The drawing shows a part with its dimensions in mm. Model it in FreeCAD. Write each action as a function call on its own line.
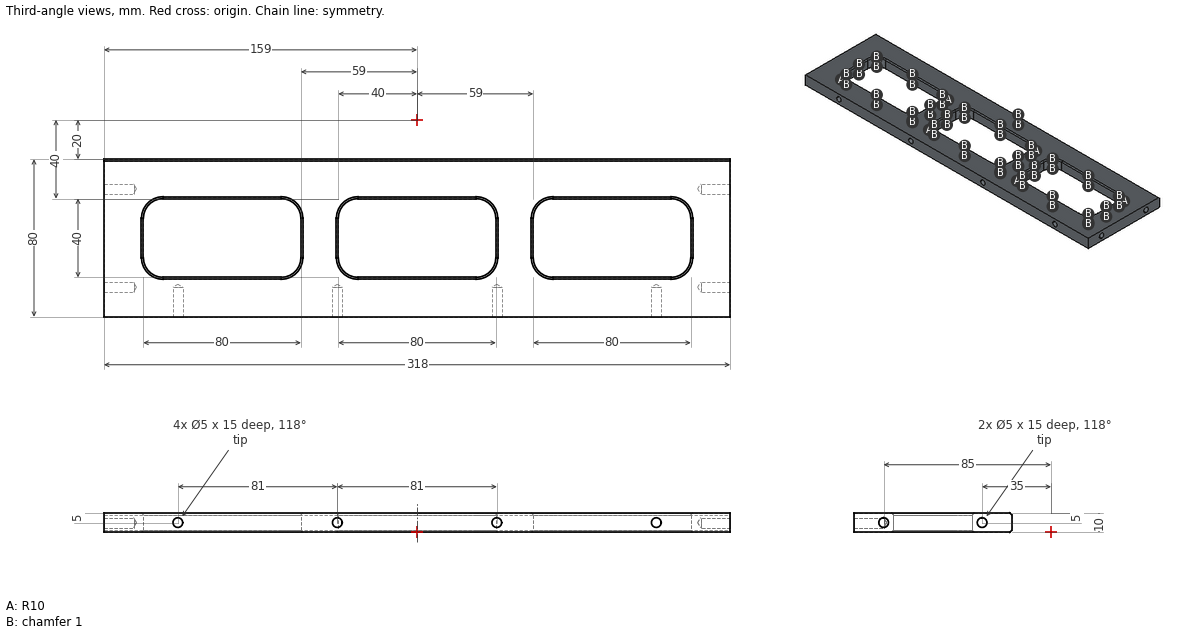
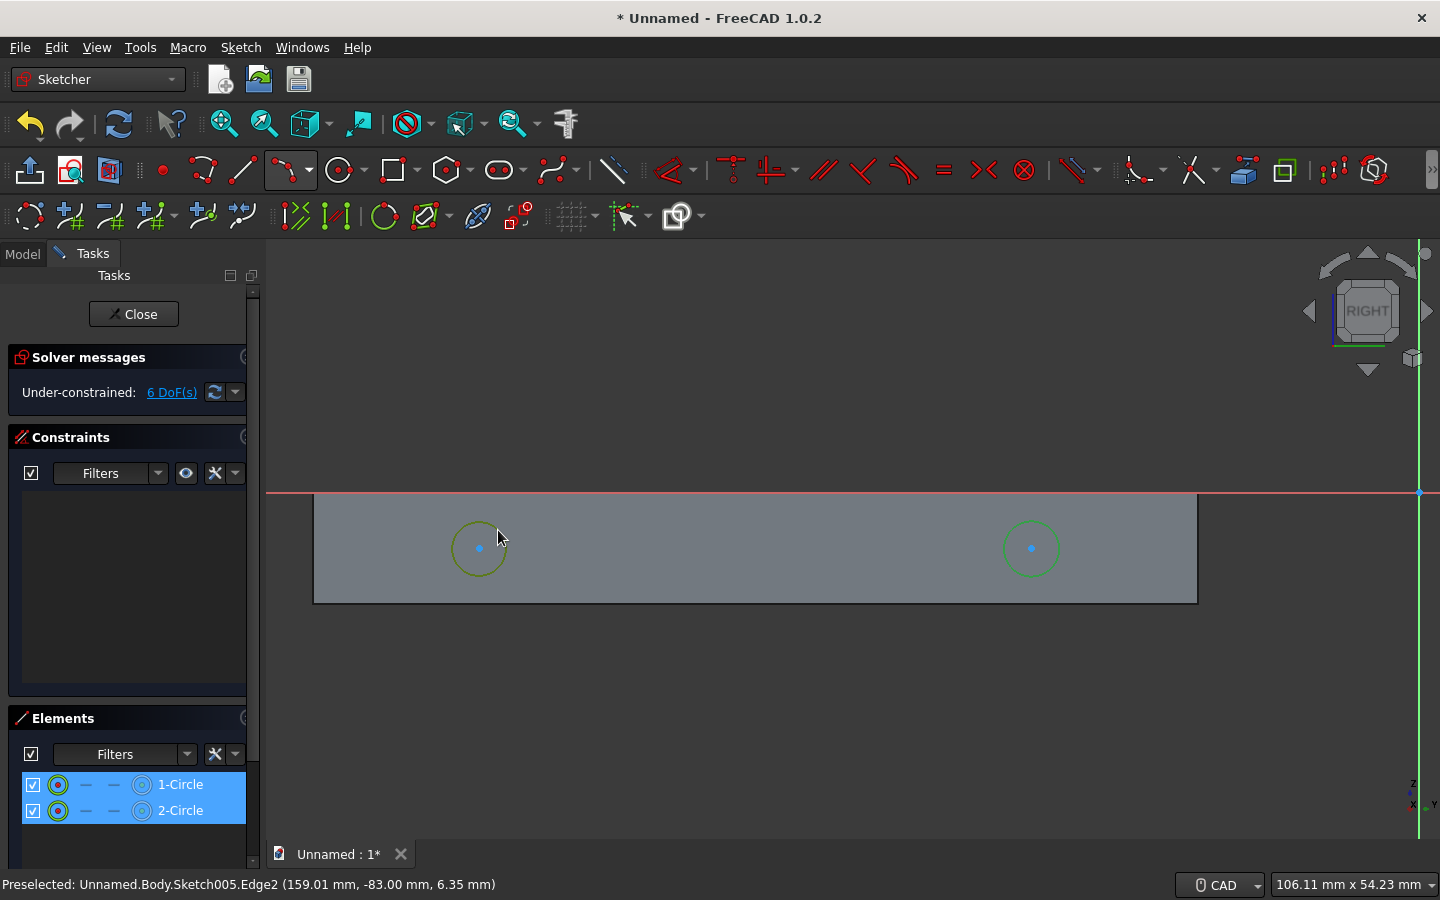
key(e)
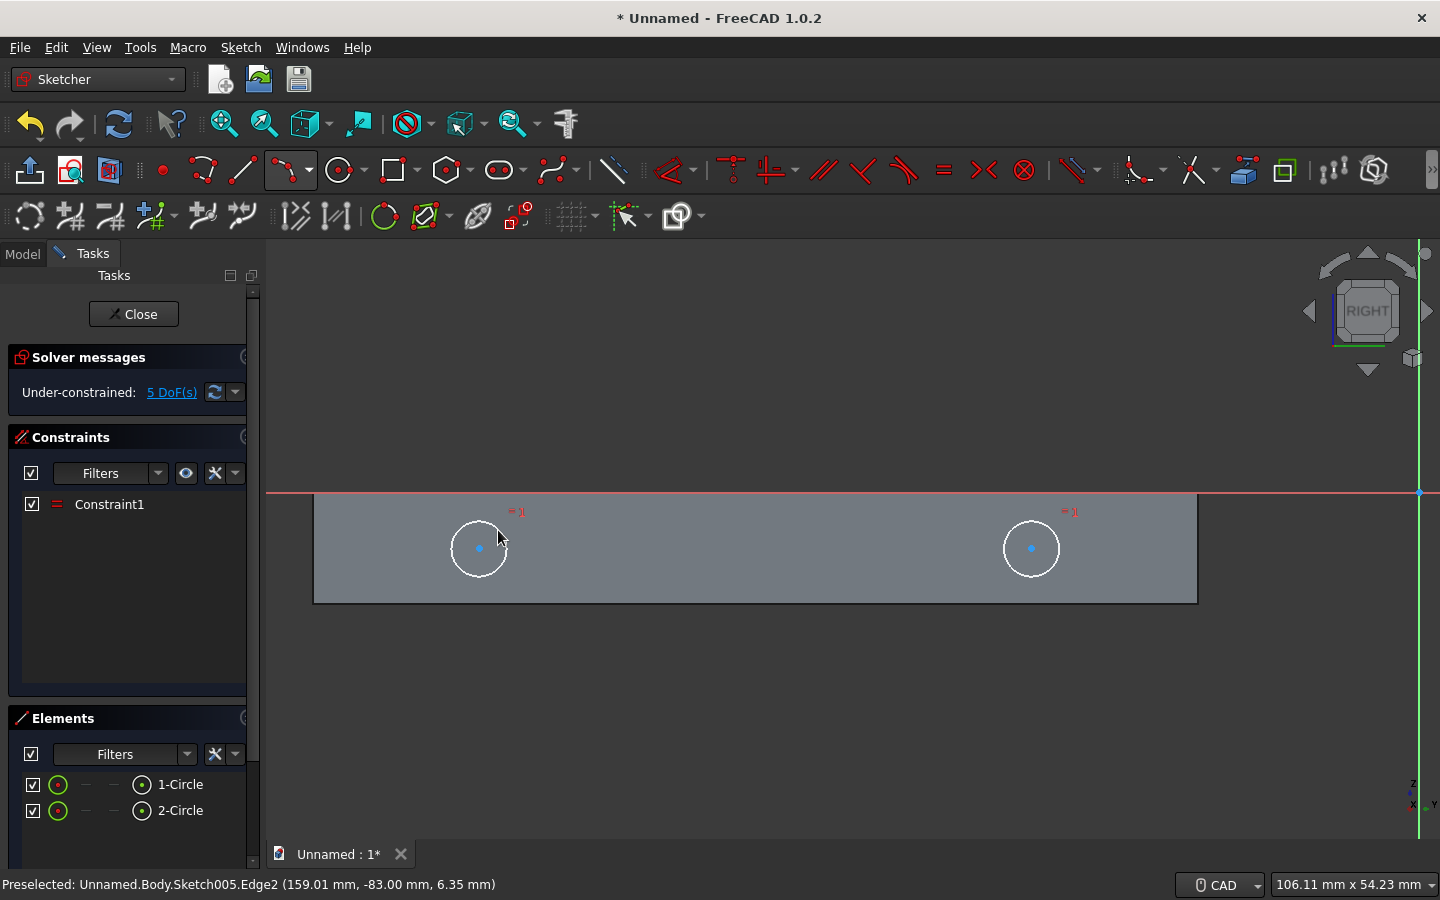
click(668, 170)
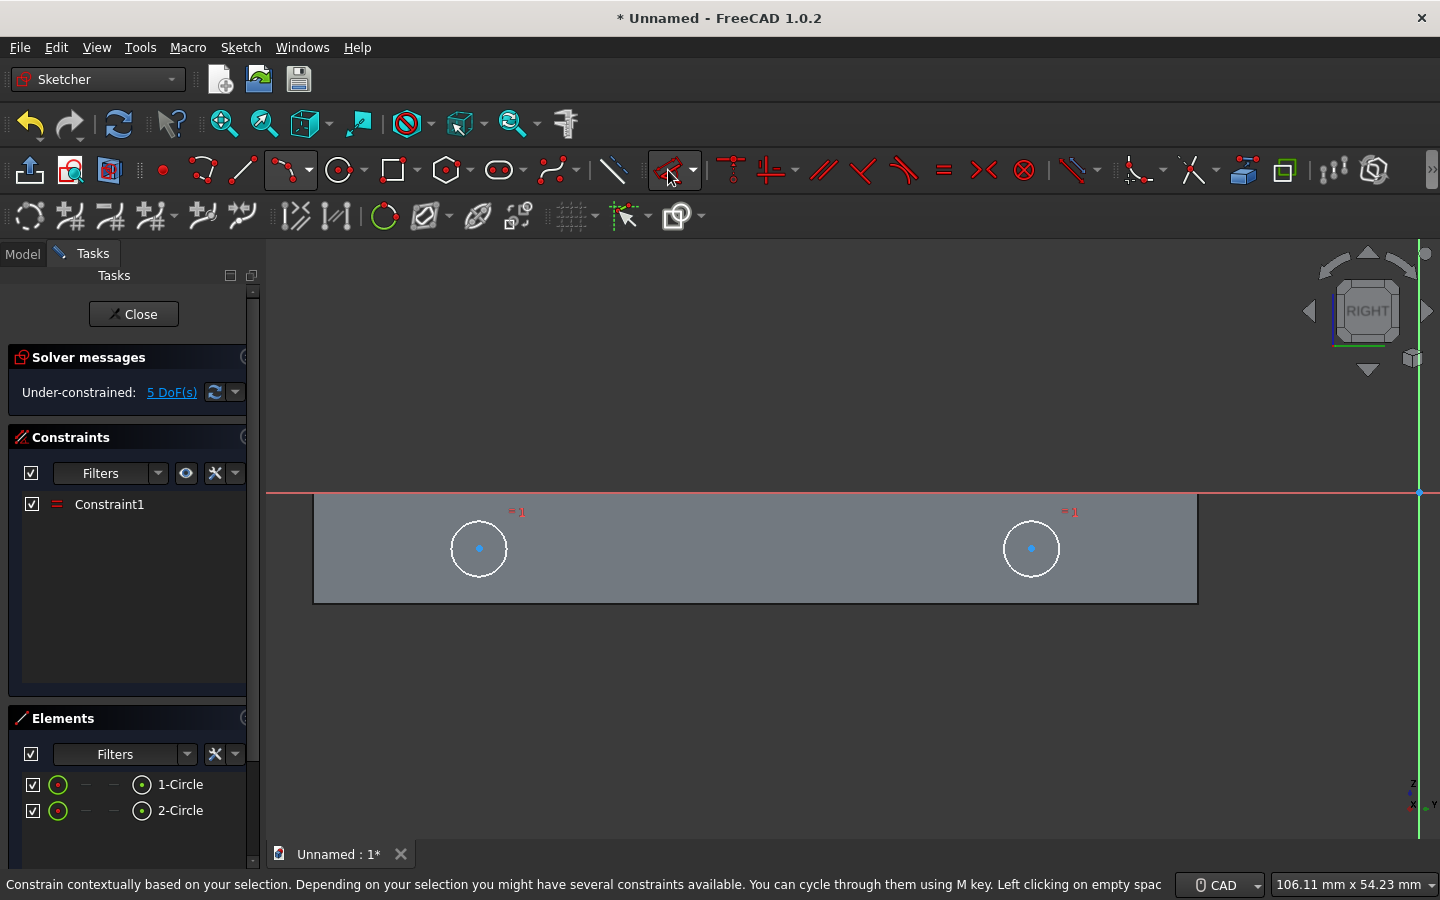
click(1051, 529)
click(1073, 506)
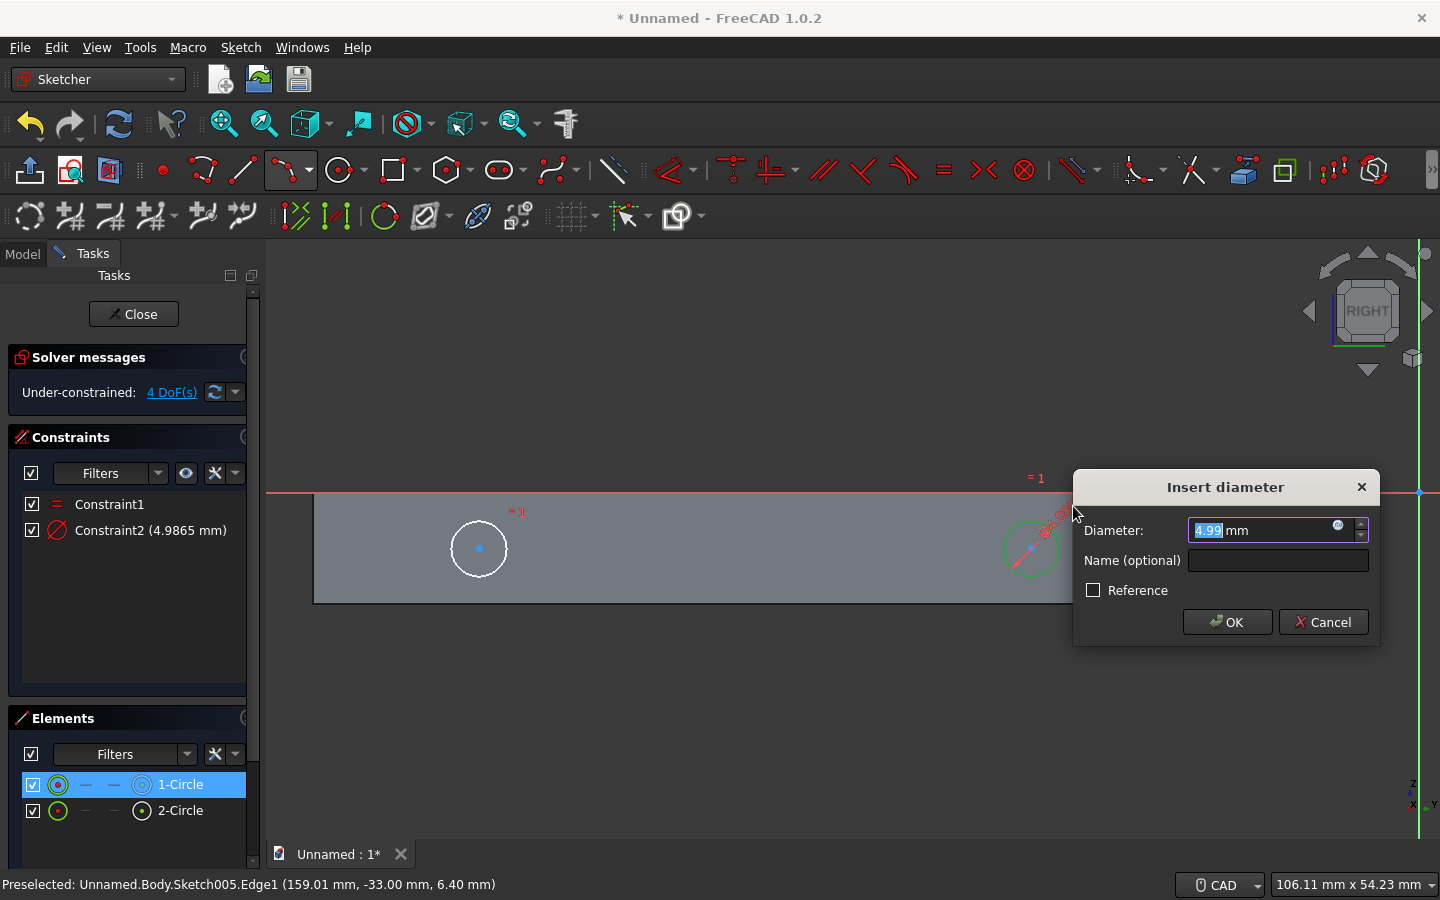
text(5)
key(Return)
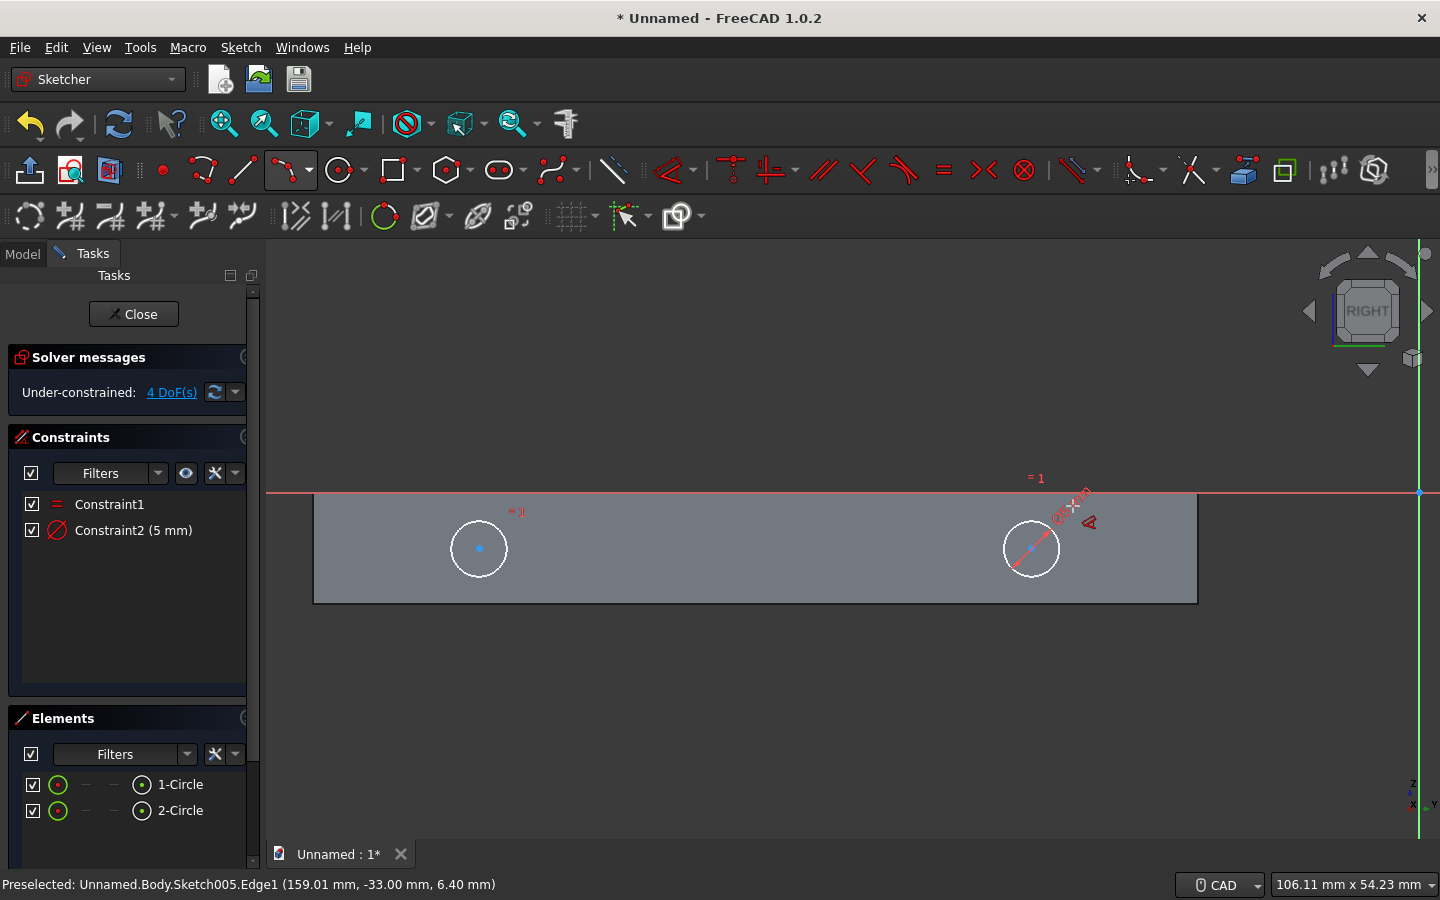
click(1032, 549)
click(998, 521)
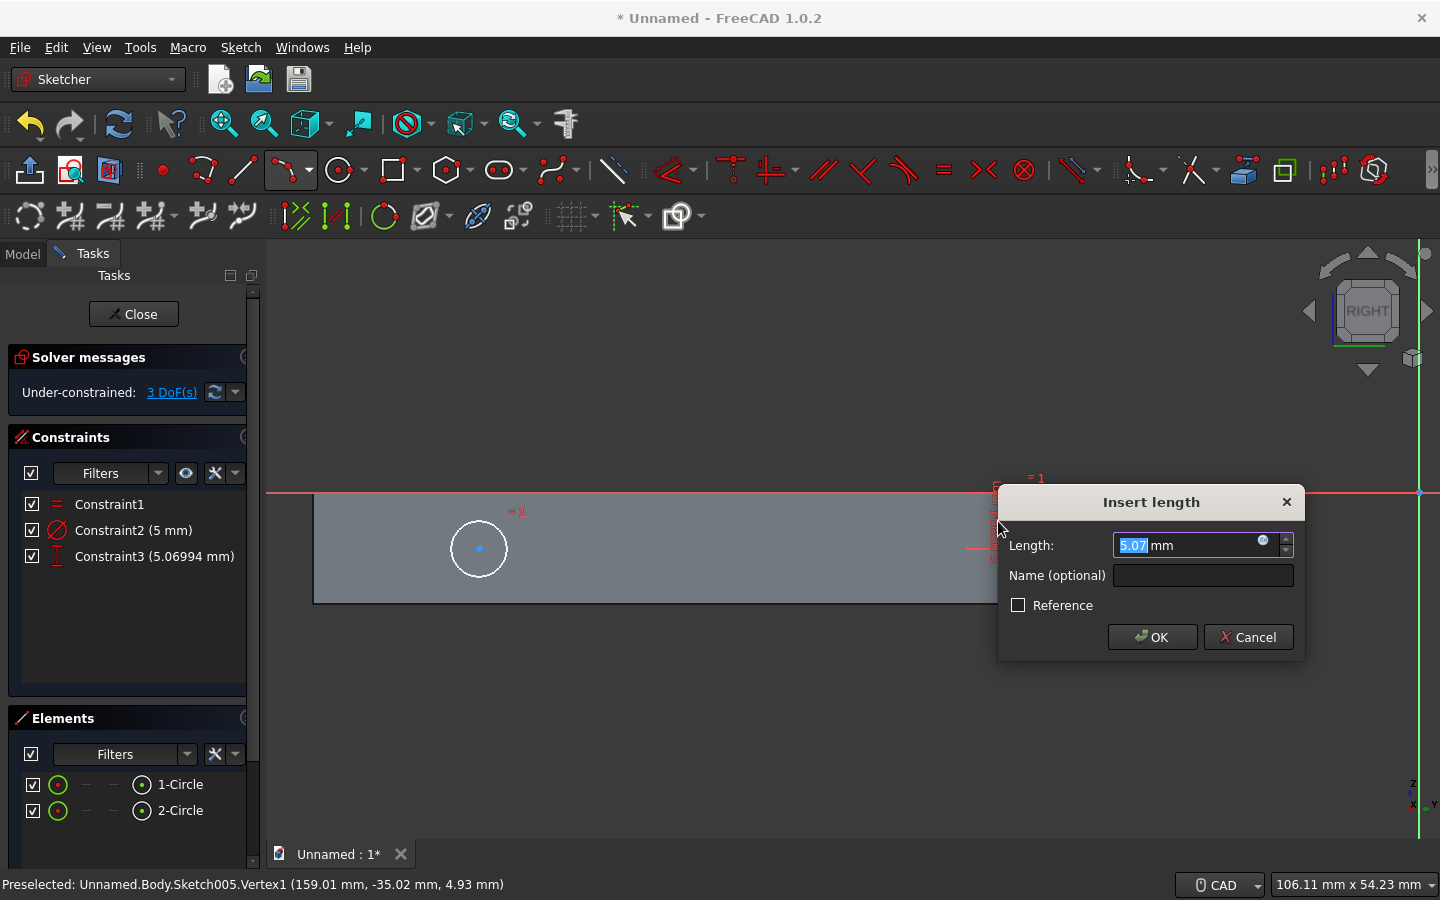
text(5)
key(Return)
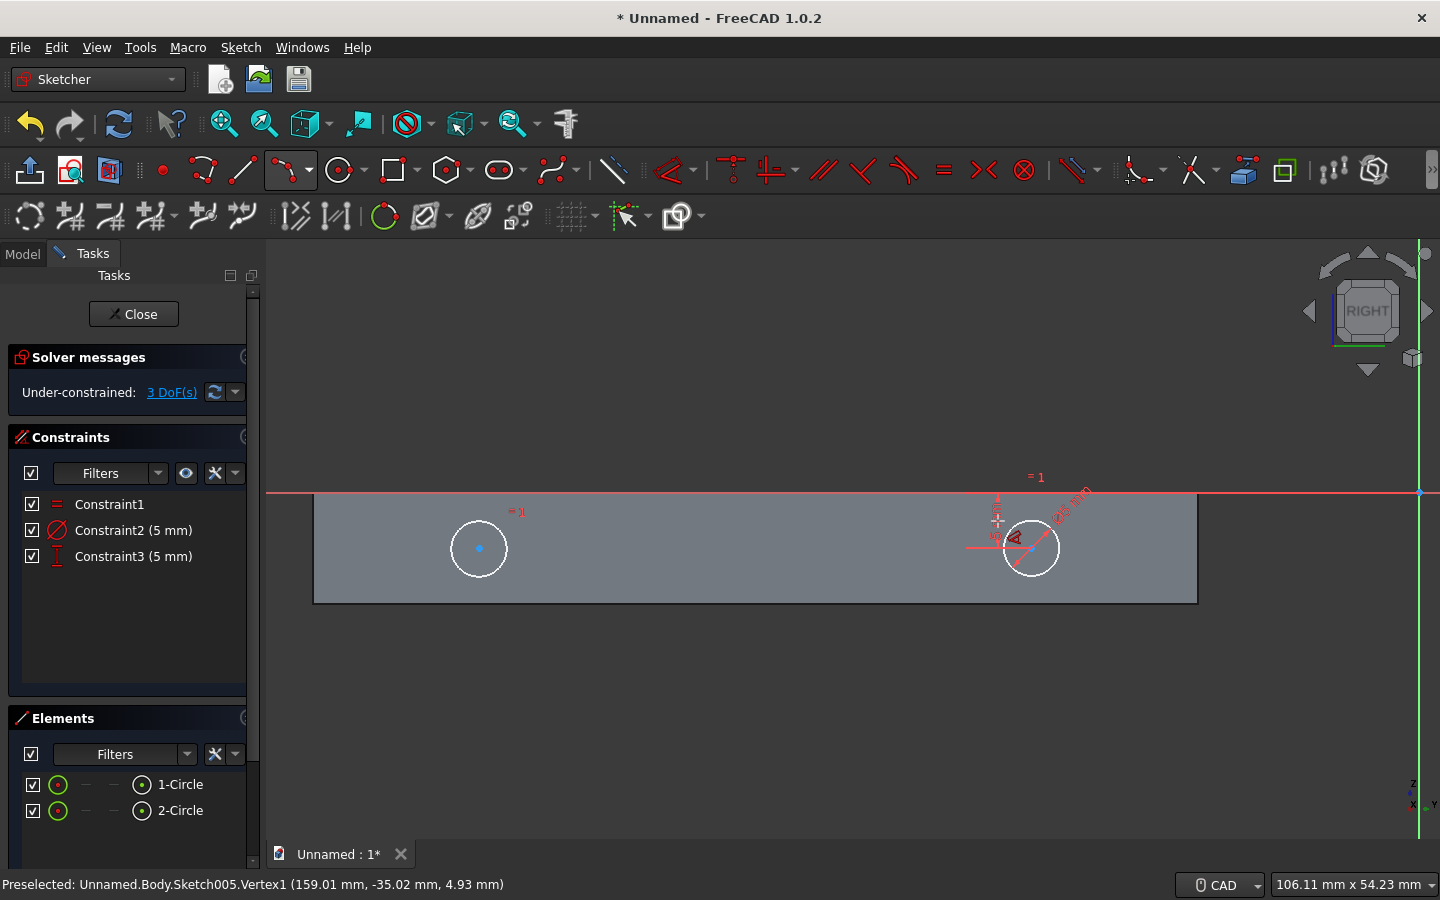
click(479, 549)
click(445, 521)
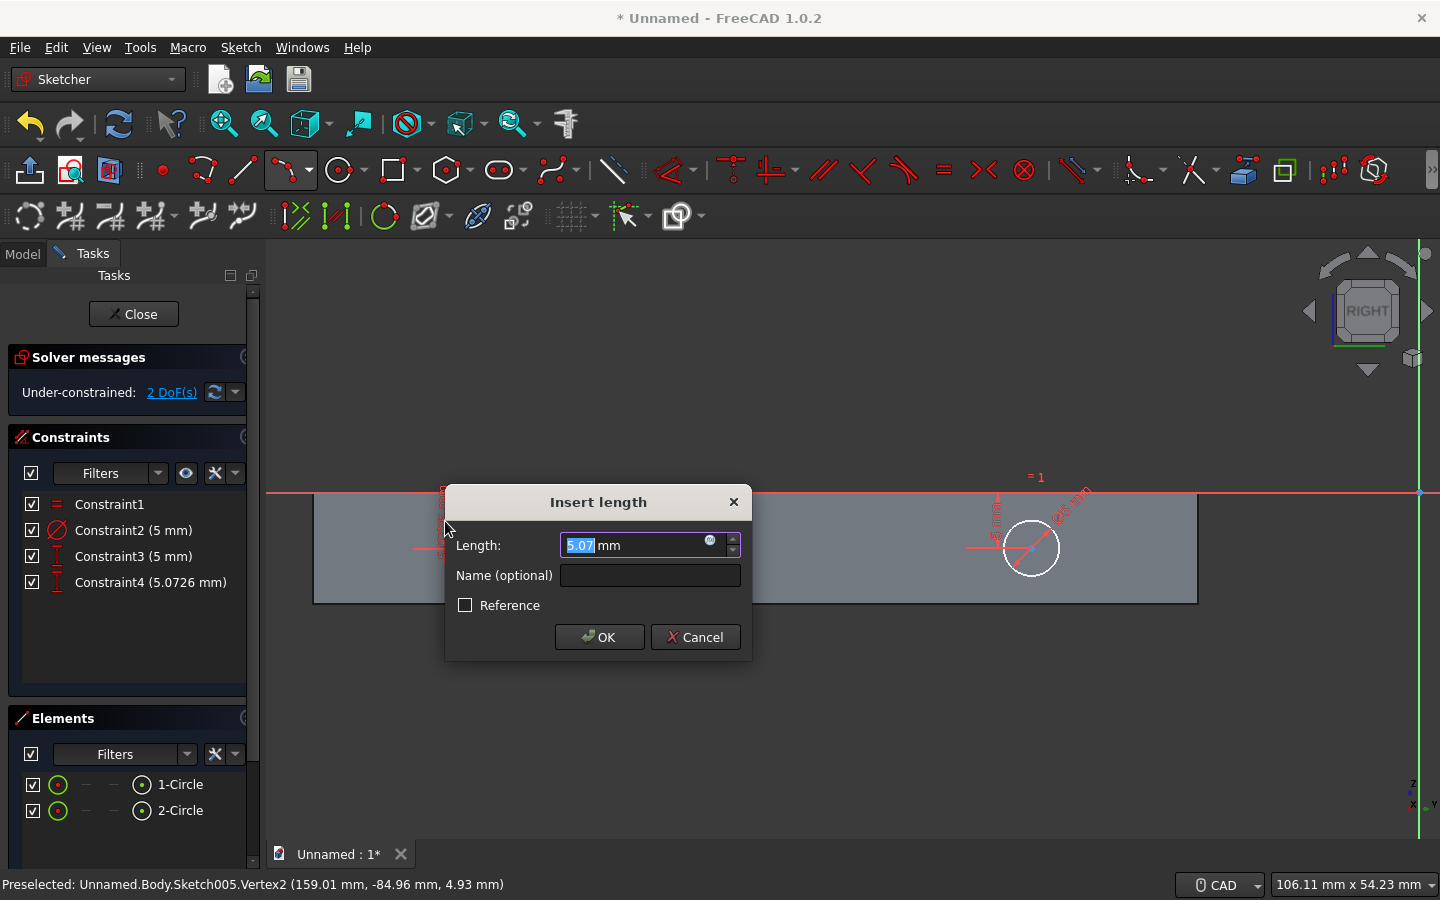
text(5)
key(Return)